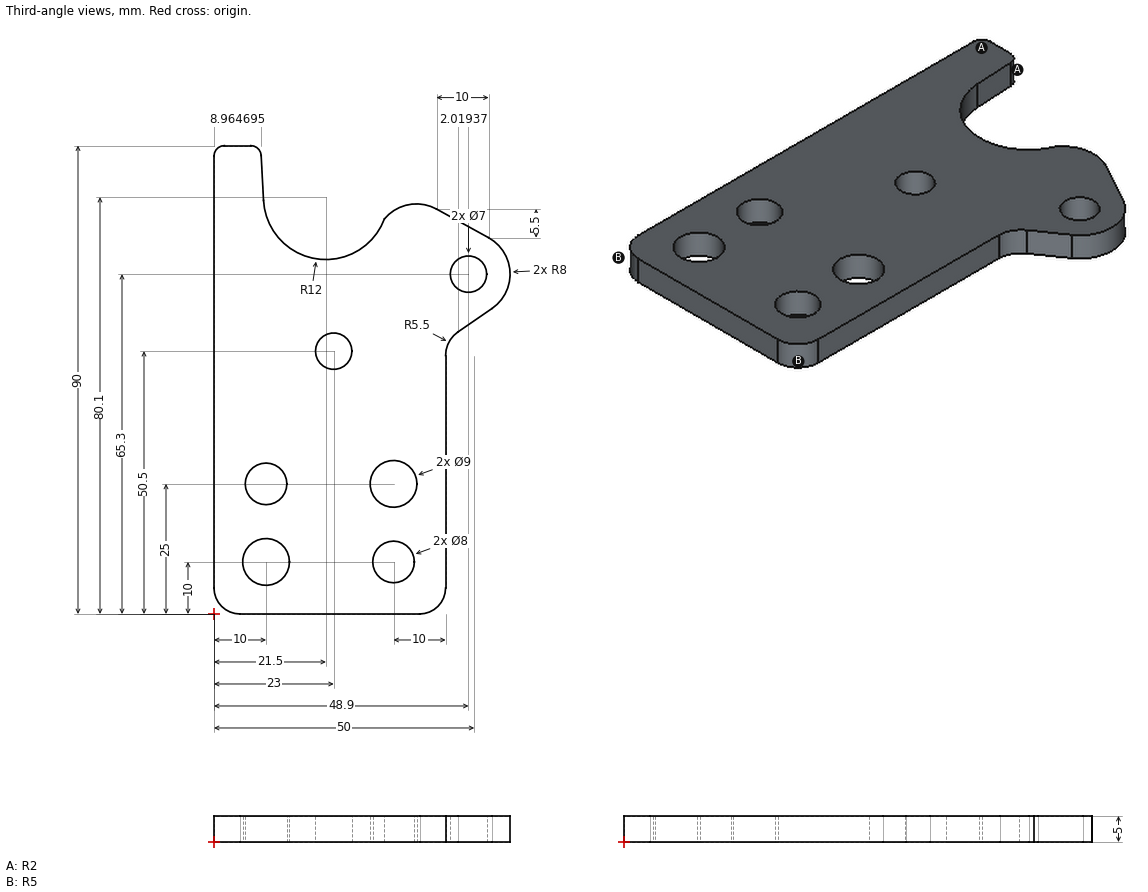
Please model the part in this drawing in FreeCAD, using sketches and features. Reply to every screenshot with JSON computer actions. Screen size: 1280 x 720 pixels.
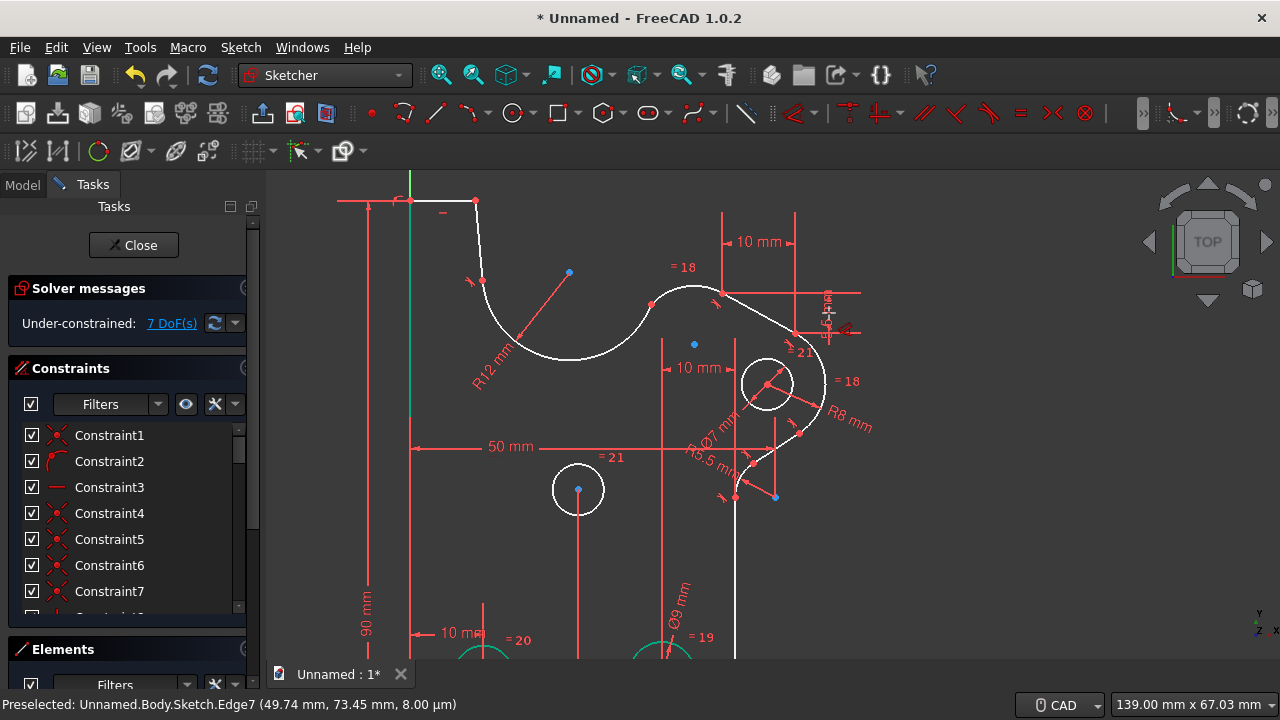
{"action": "left_click", "coordinate": [767, 384]}
{"action": "left_click", "coordinate": [589, 326]}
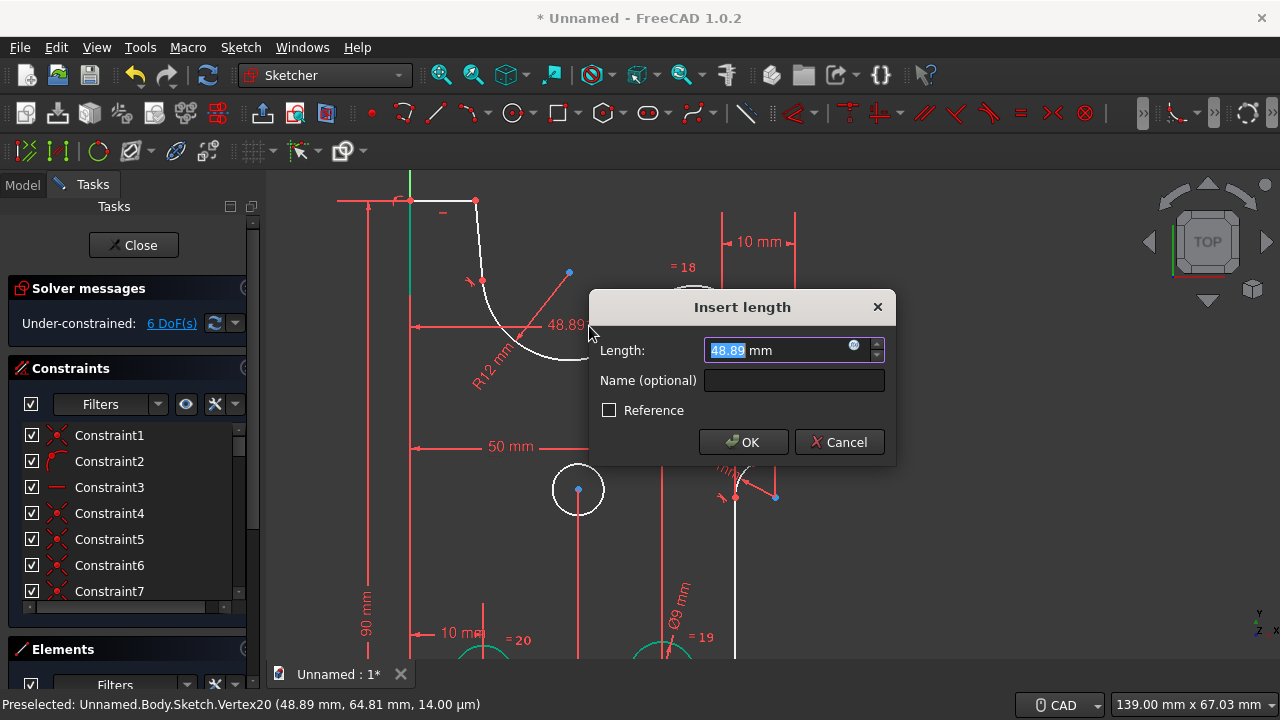
{"action": "type", "text": "48.9"}
{"action": "key", "text": "Return"}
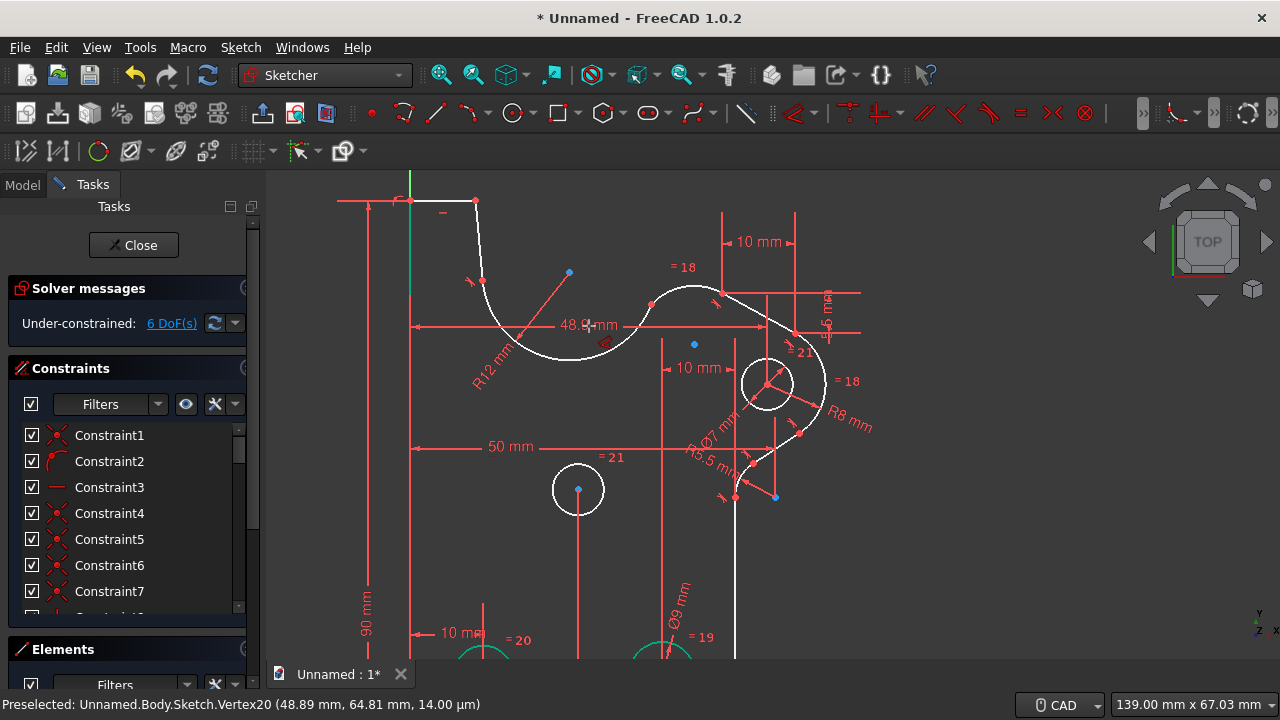
{"action": "left_click", "coordinate": [767, 384]}
{"action": "left_click", "coordinate": [376, 508]}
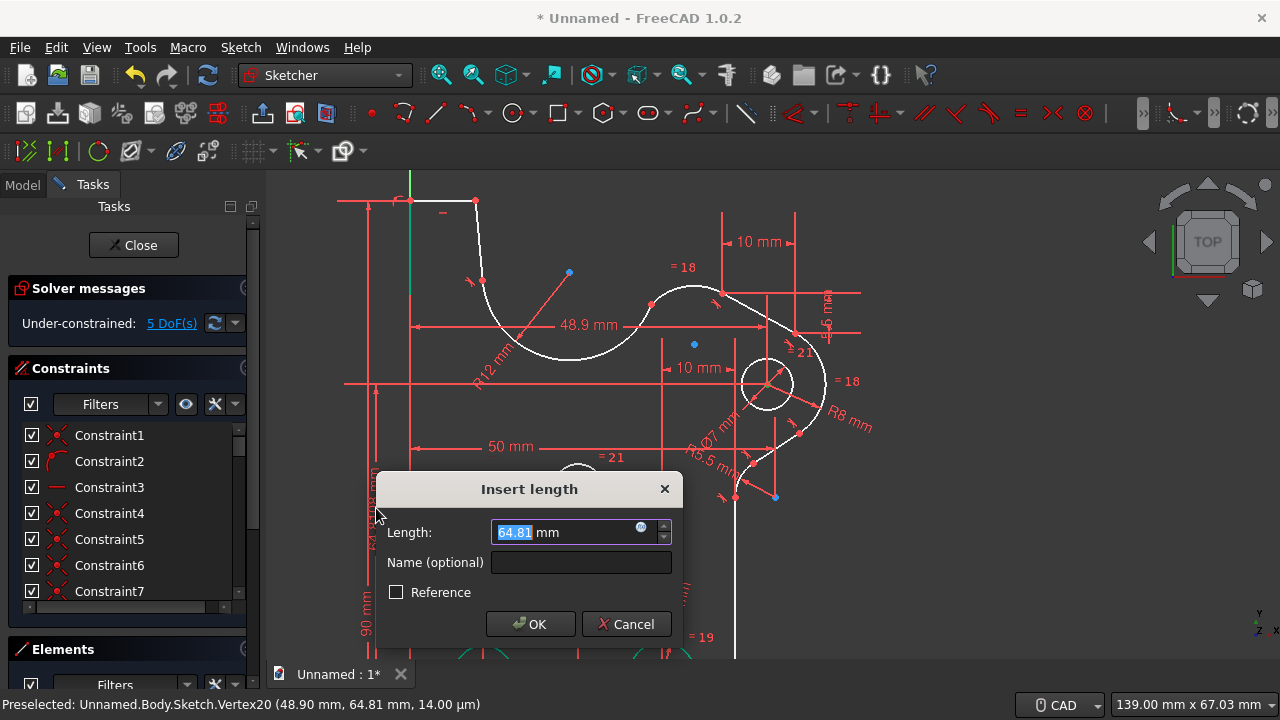
{"action": "type", "text": "65.3"}
{"action": "key", "text": "Return"}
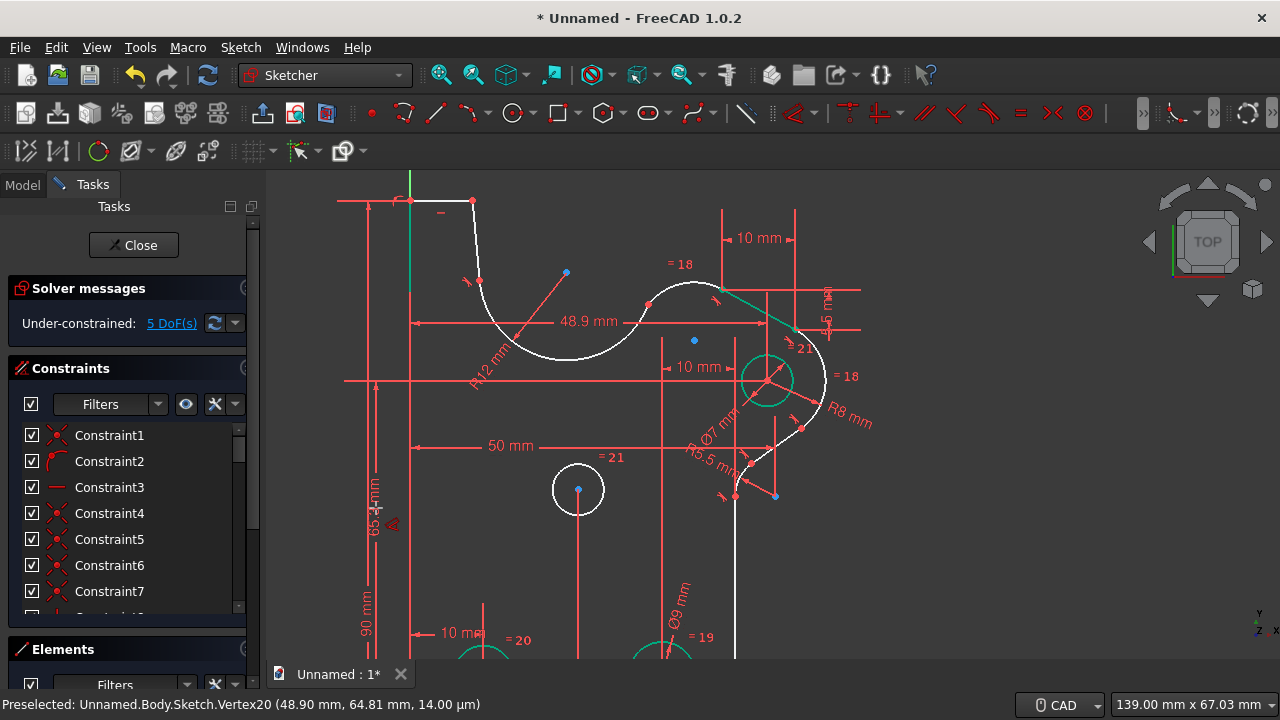
{"action": "left_click", "coordinate": [578, 490]}
{"action": "left_click", "coordinate": [376, 560]}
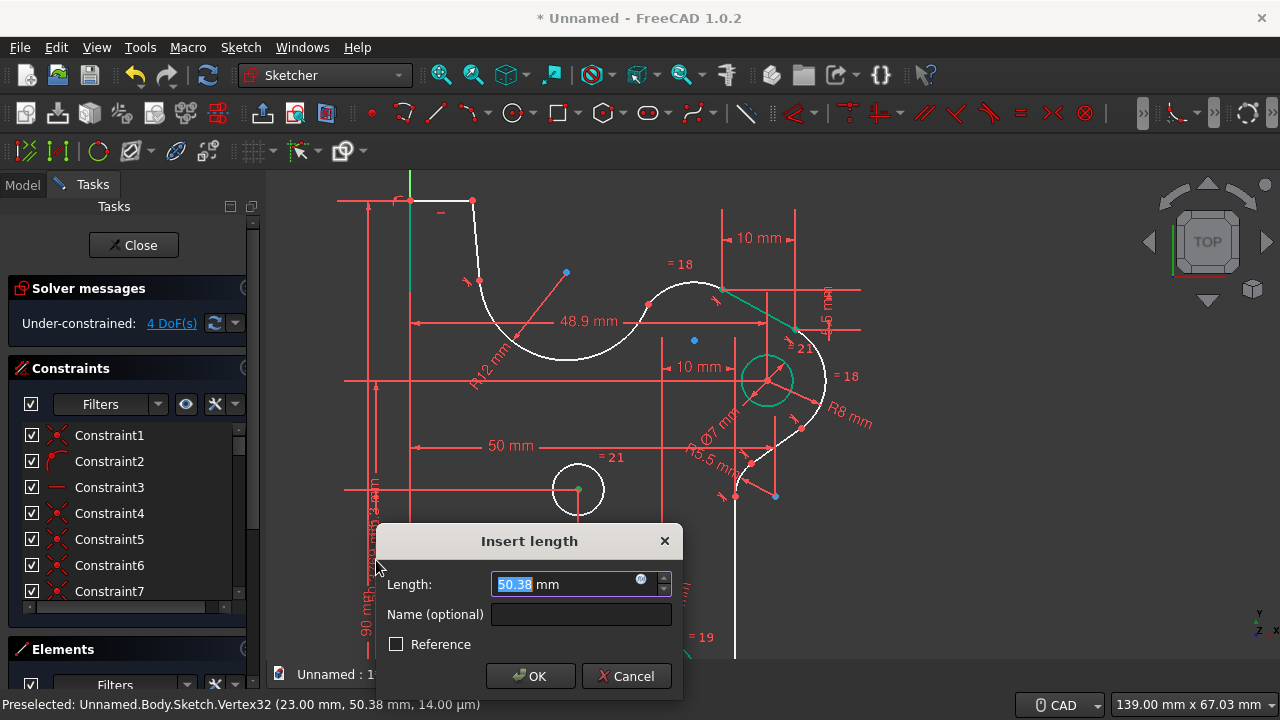
{"action": "type", "text": "50.5"}
{"action": "key", "text": "Return"}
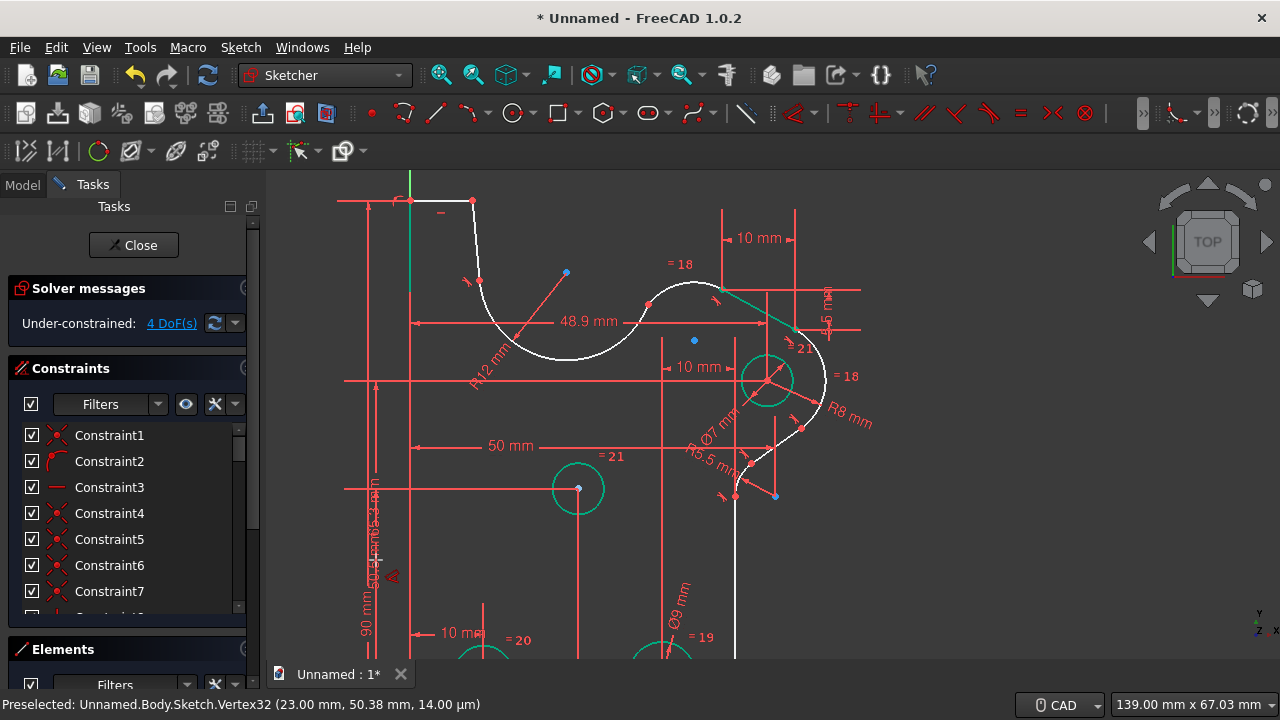
{"action": "left_click", "coordinate": [567, 273]}
{"action": "left_click", "coordinate": [453, 239]}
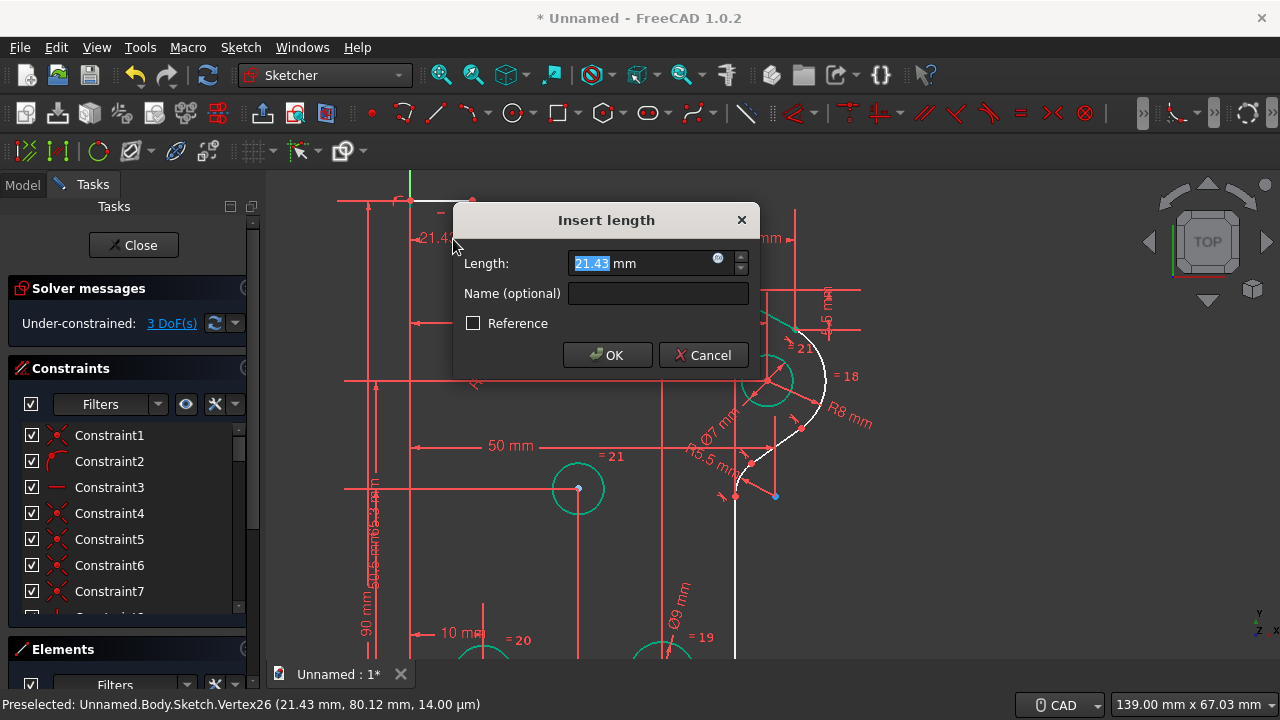
{"action": "type", "text": "21.5"}
{"action": "key", "text": "Return"}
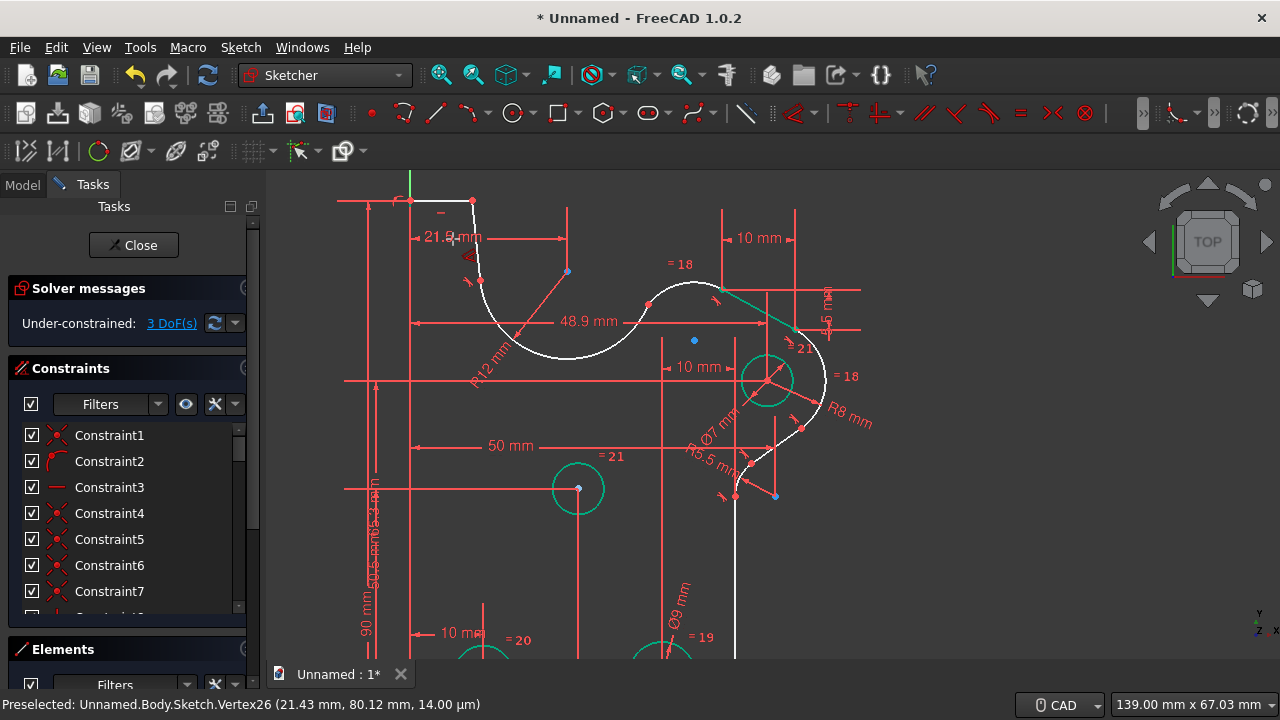
{"action": "left_click", "coordinate": [567, 271]}
{"action": "left_click", "coordinate": [376, 451]}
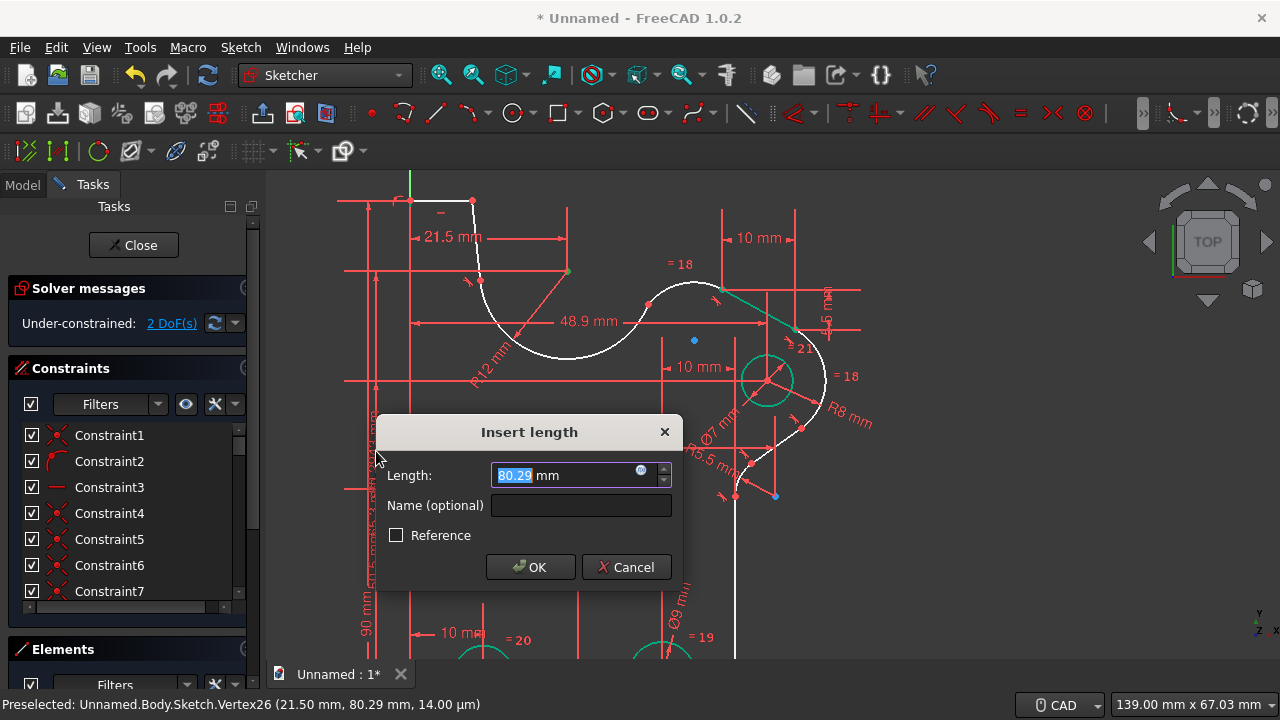
{"action": "type", "text": "80.1"}
{"action": "key", "text": "Return"}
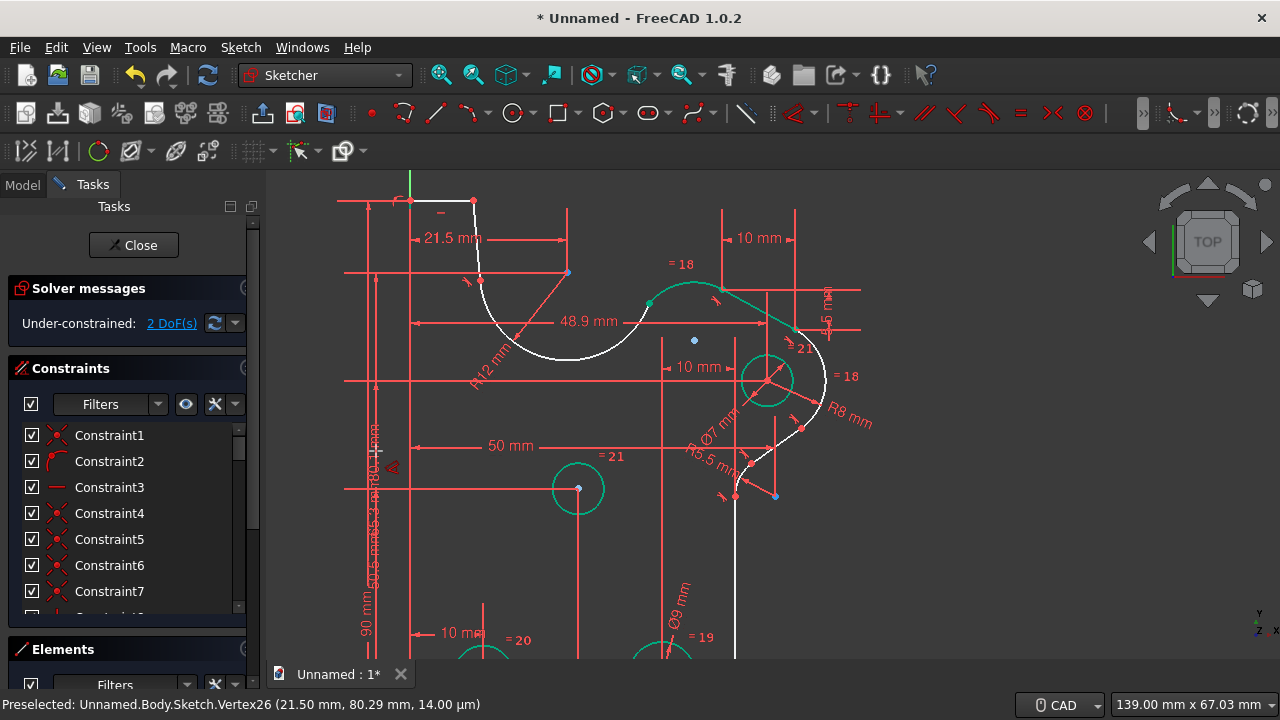
{"action": "left_click", "coordinate": [454, 201]}
{"action": "left_click", "coordinate": [442, 283]}